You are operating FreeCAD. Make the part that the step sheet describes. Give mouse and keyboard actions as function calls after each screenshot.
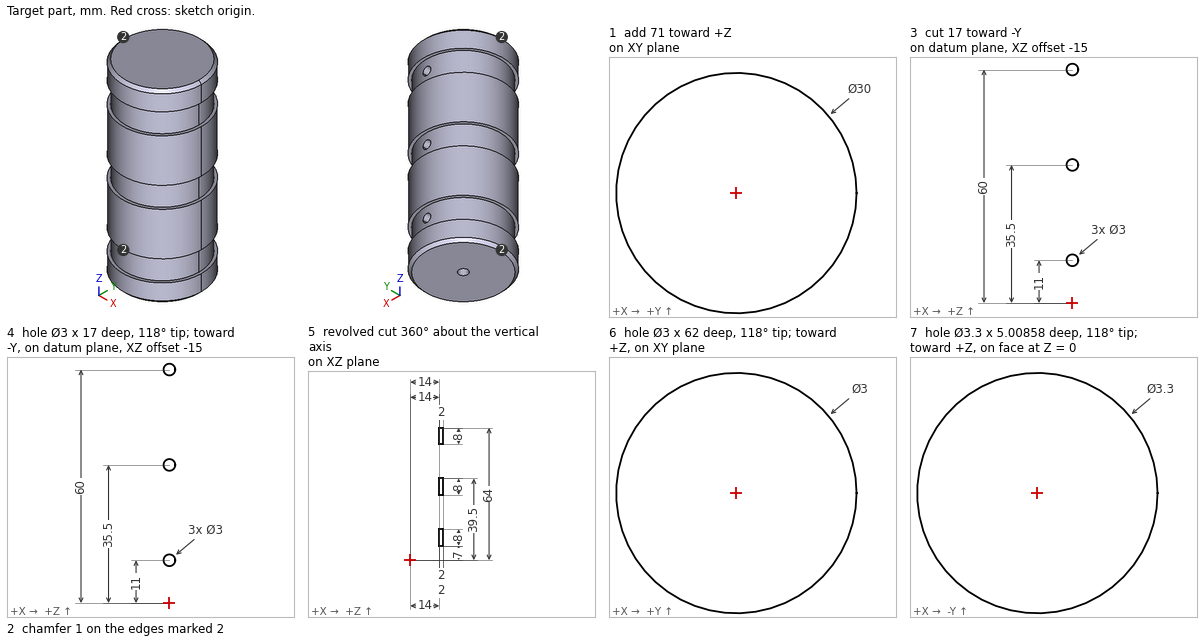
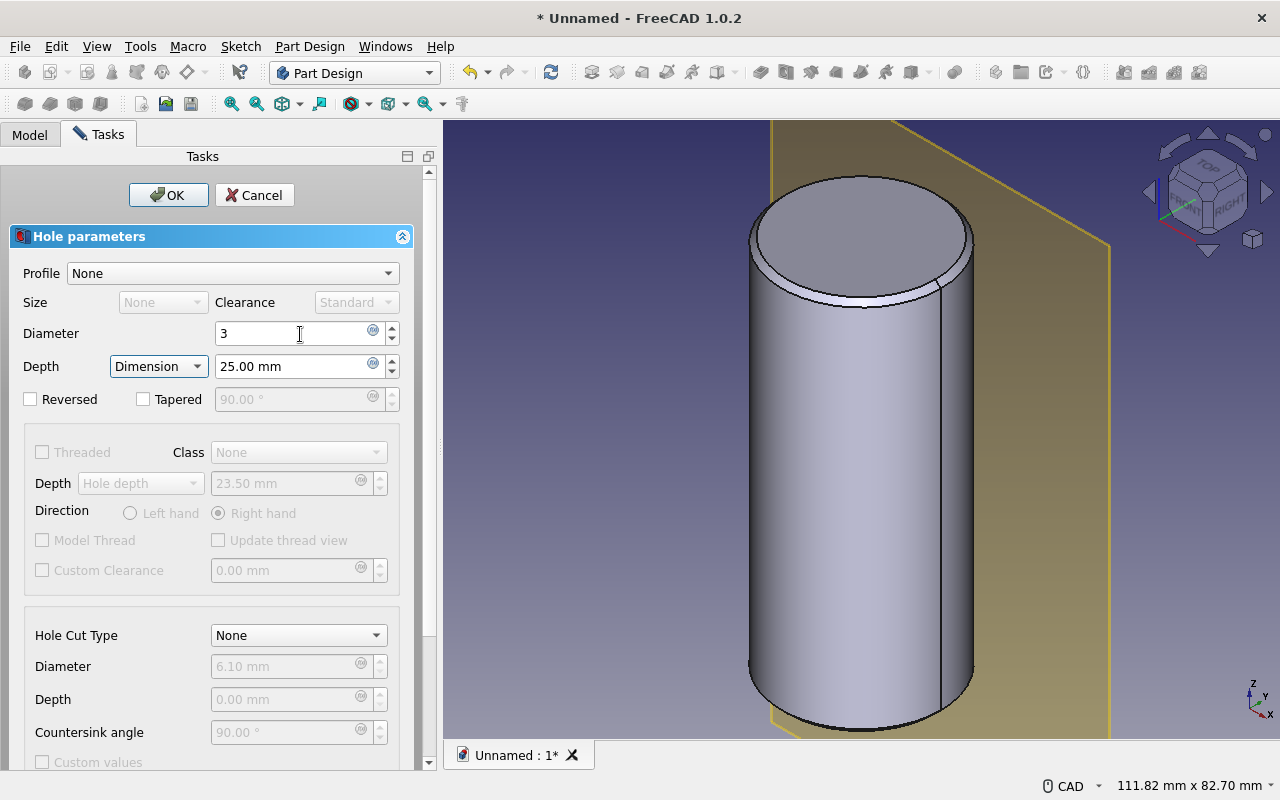
triple_click(300, 366)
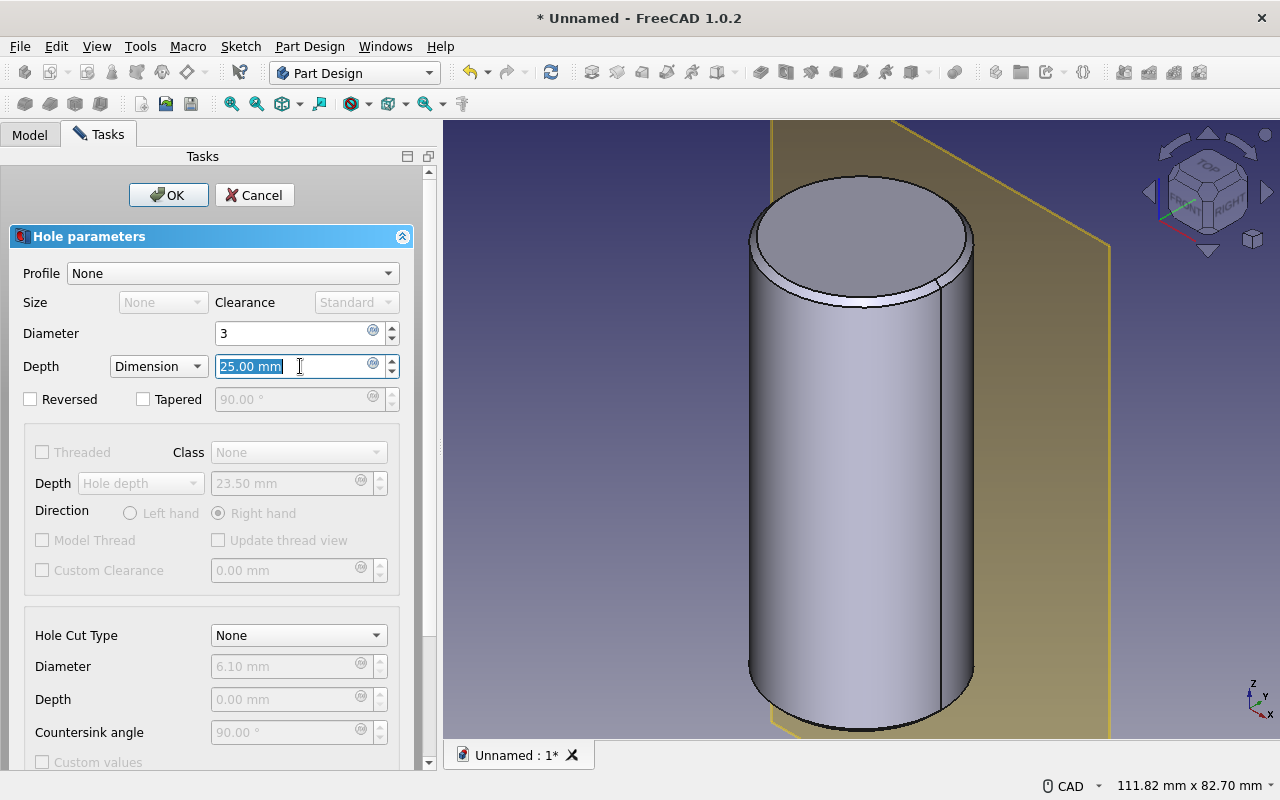
text(17)
key(Tab)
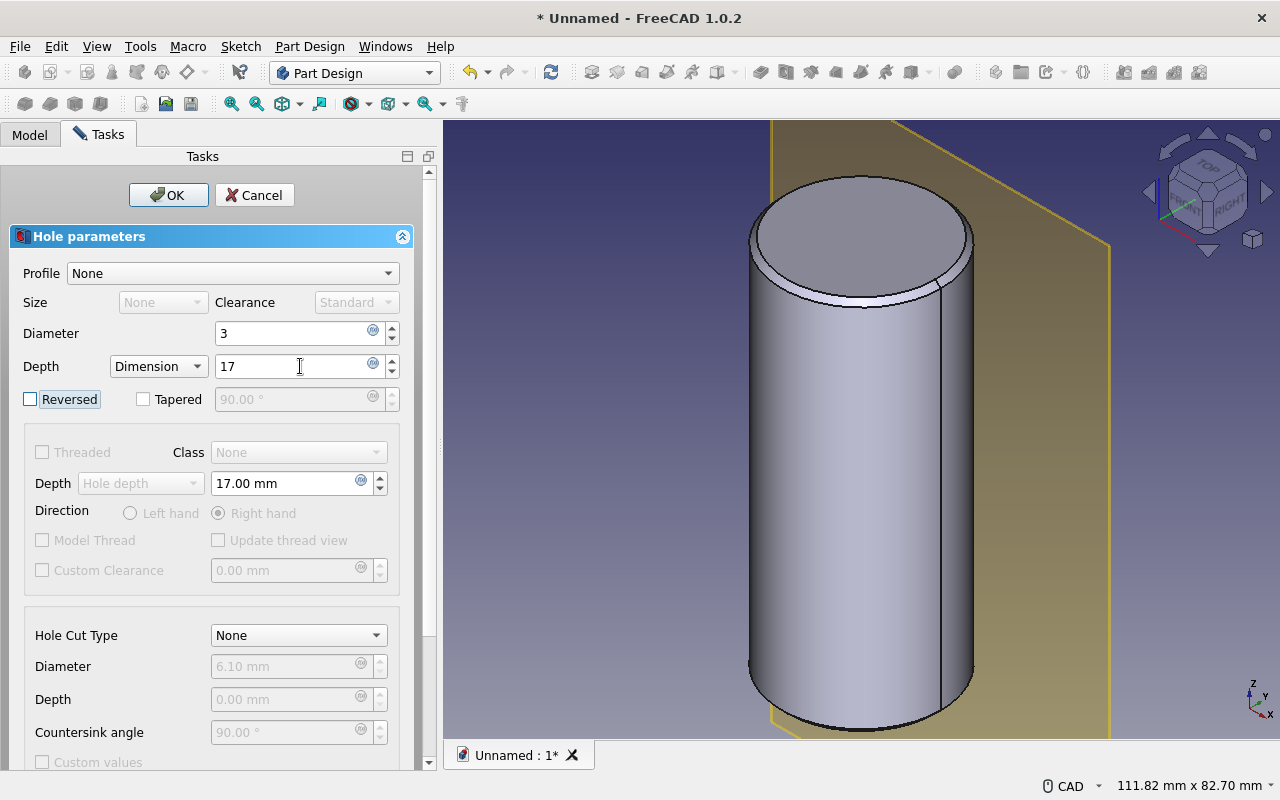
click(31, 399)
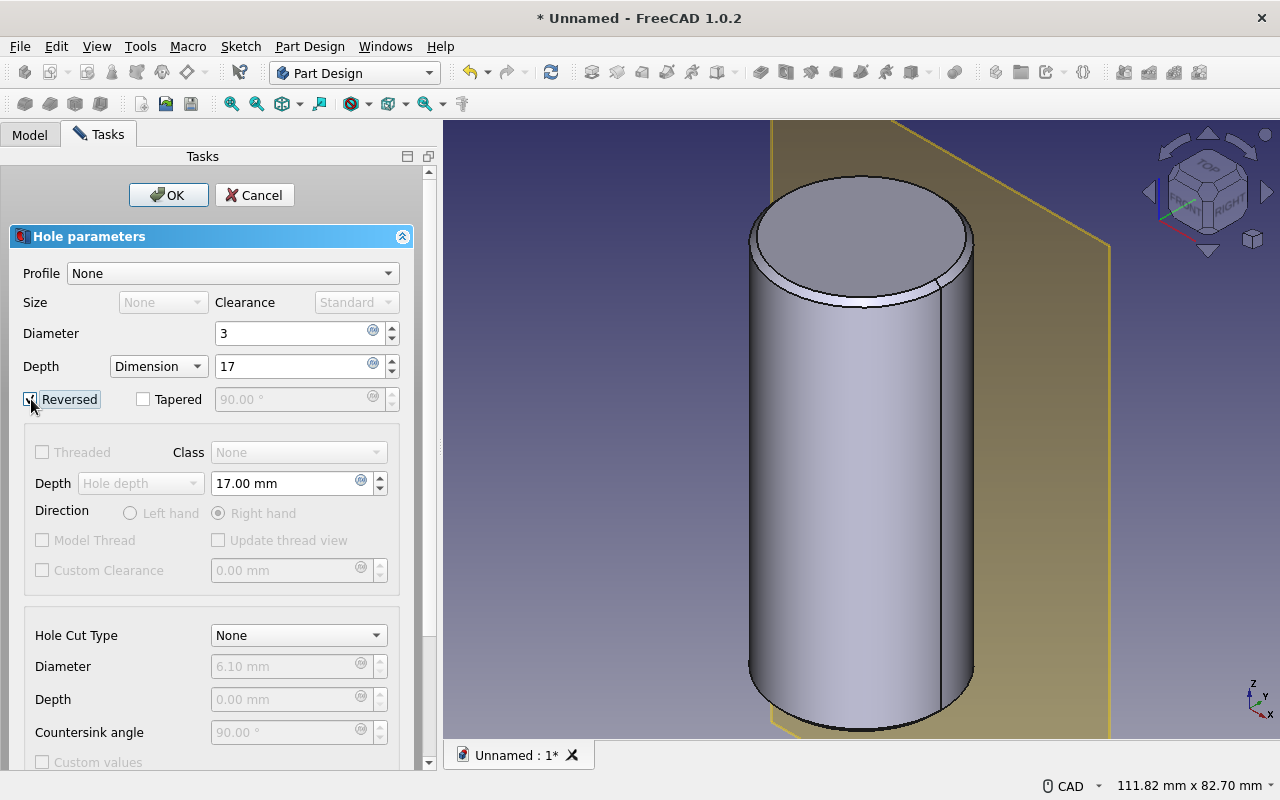
click(169, 195)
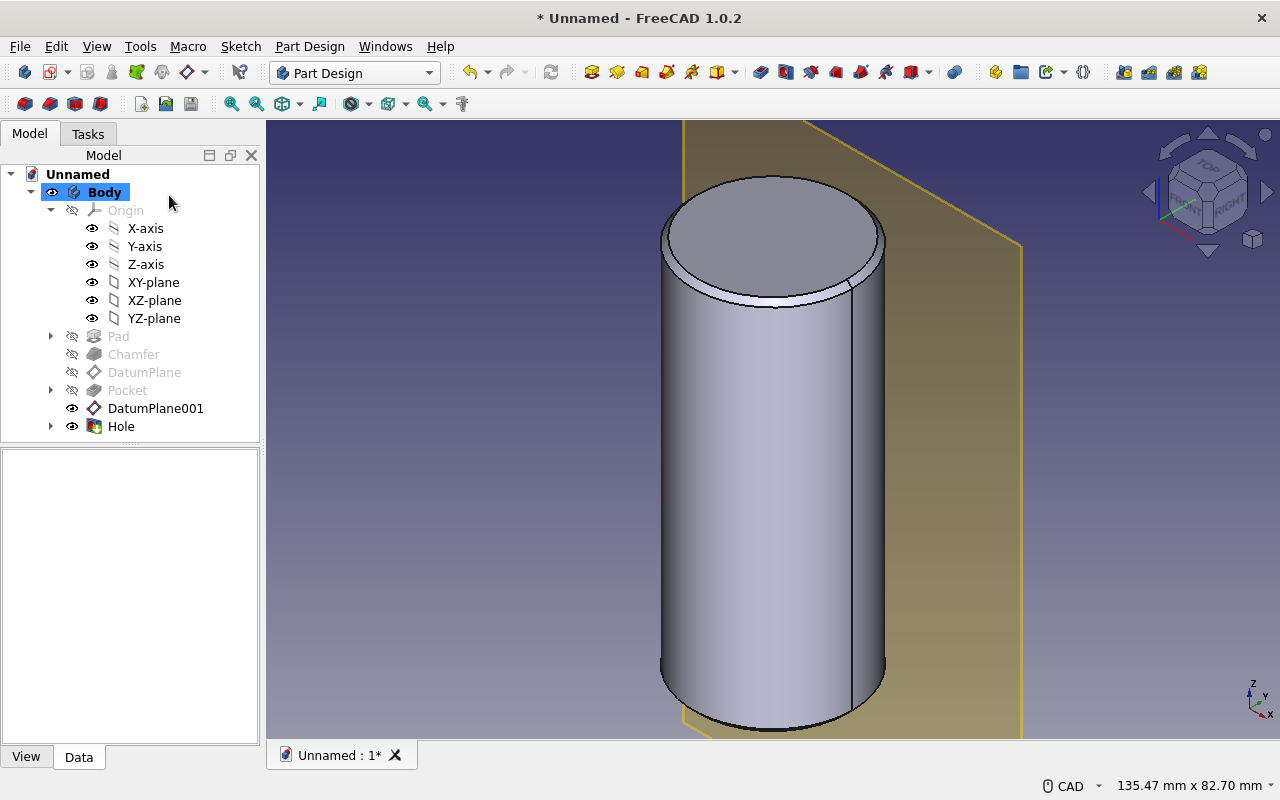
click(117, 408)
key(space)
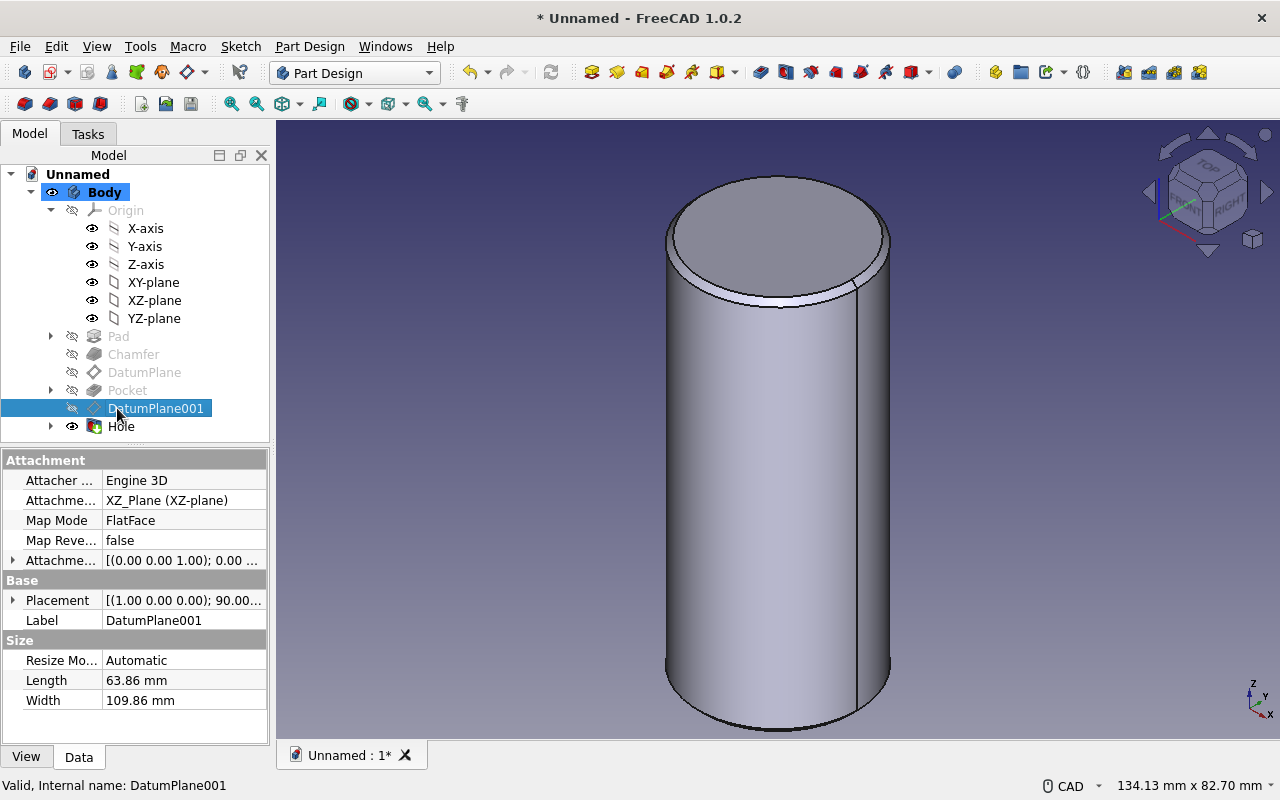
click(232, 104)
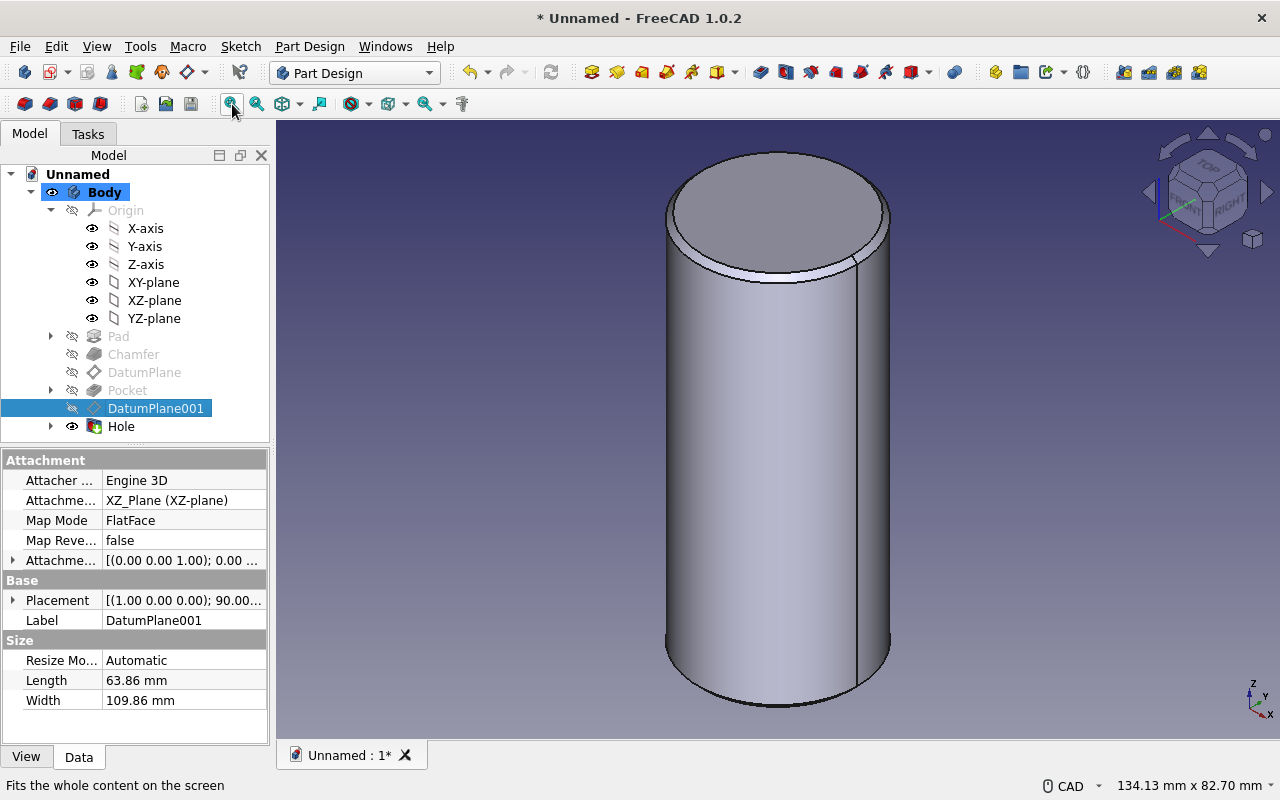
click(316, 699)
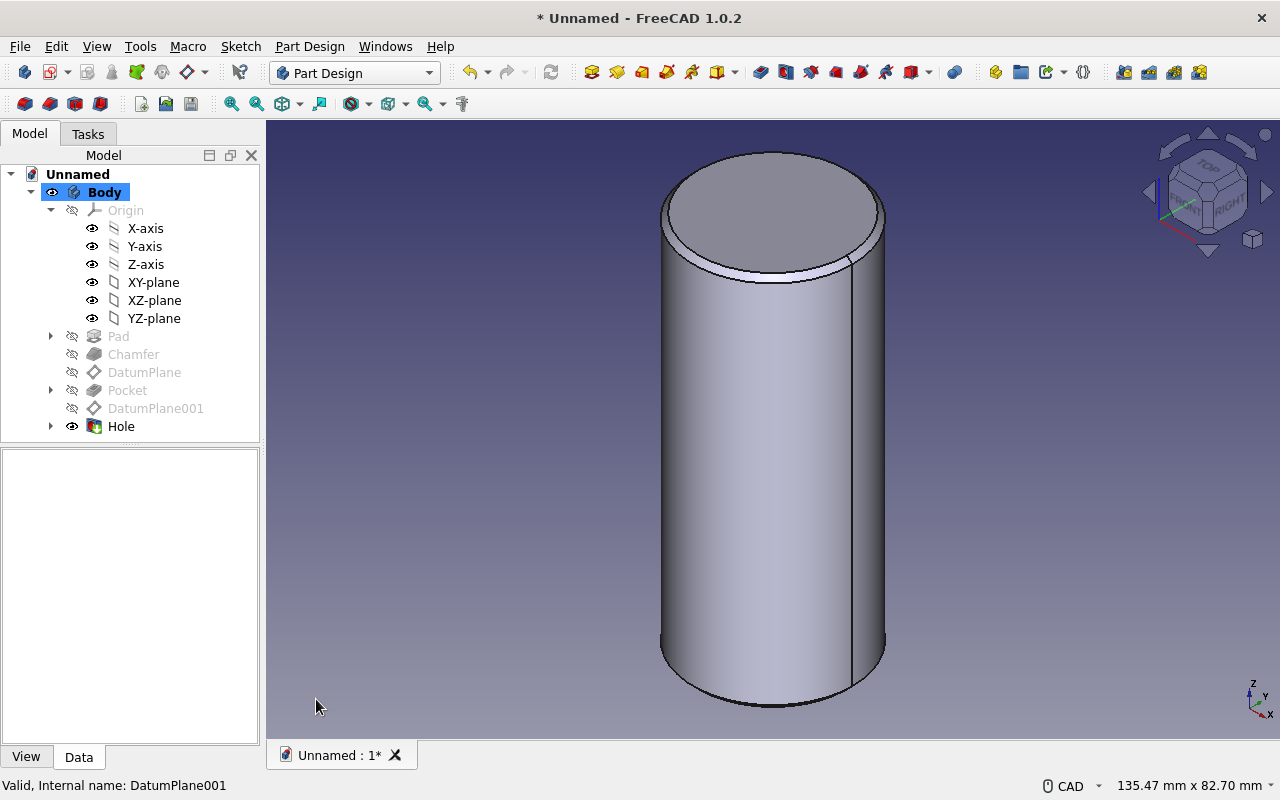
click(50, 72)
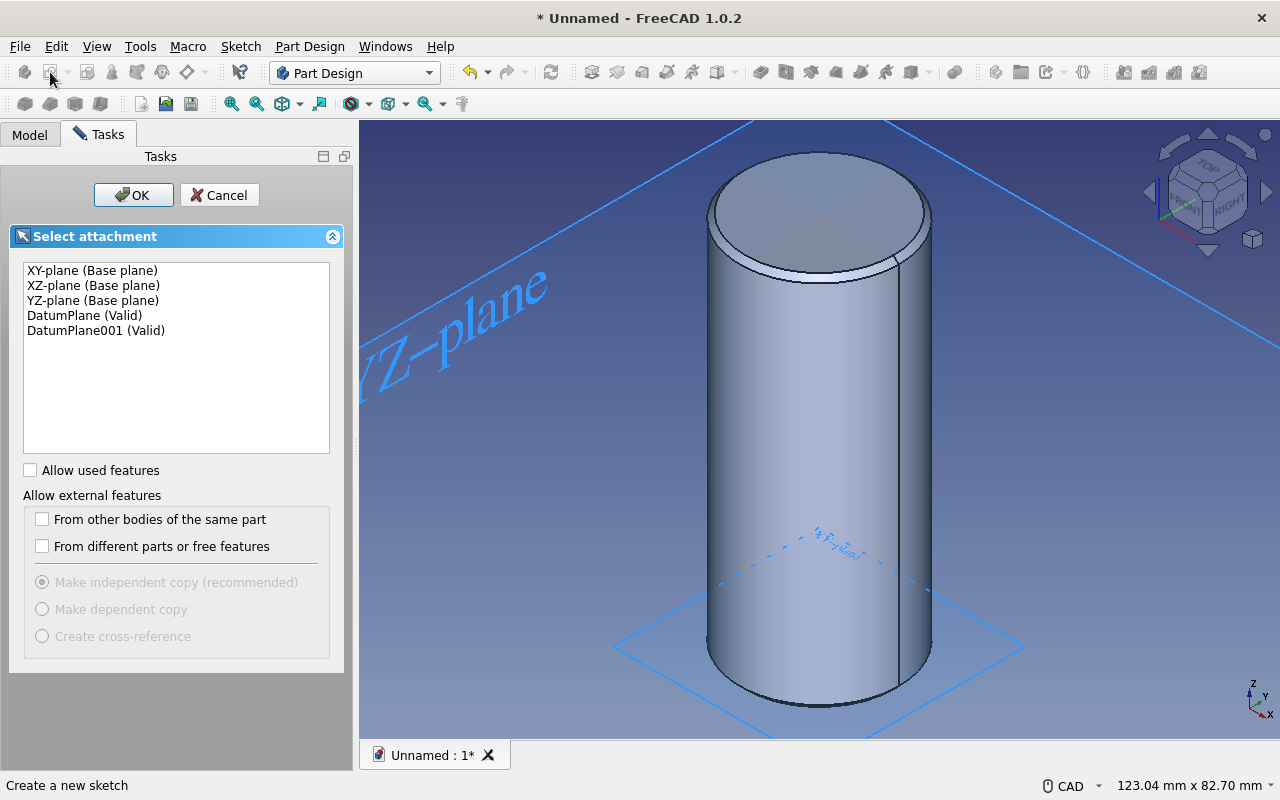
click(84, 286)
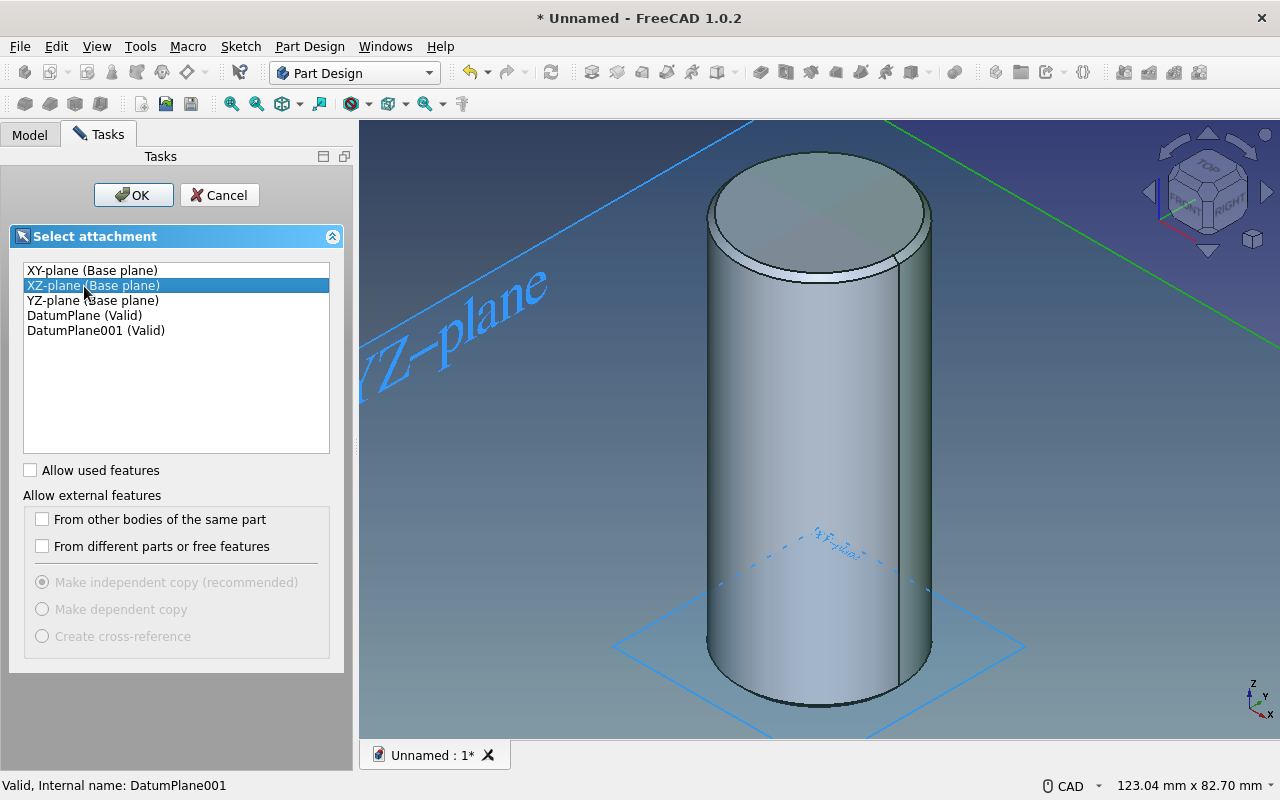
click(134, 195)